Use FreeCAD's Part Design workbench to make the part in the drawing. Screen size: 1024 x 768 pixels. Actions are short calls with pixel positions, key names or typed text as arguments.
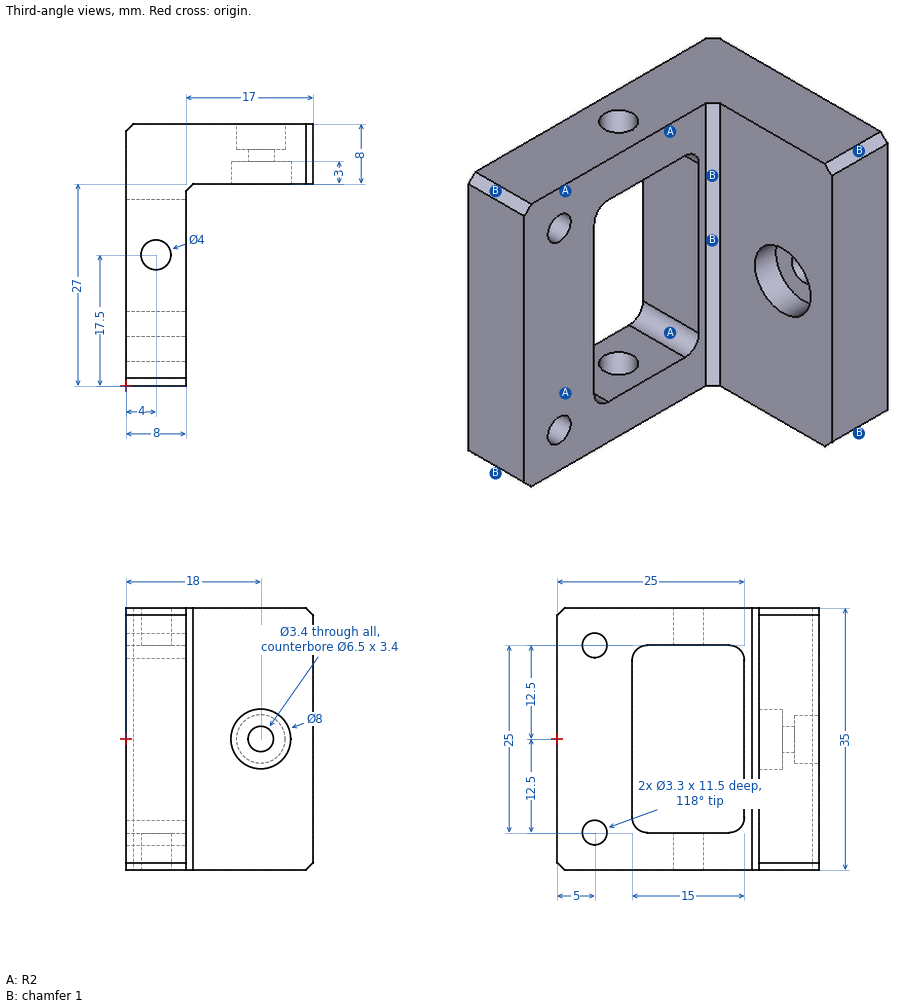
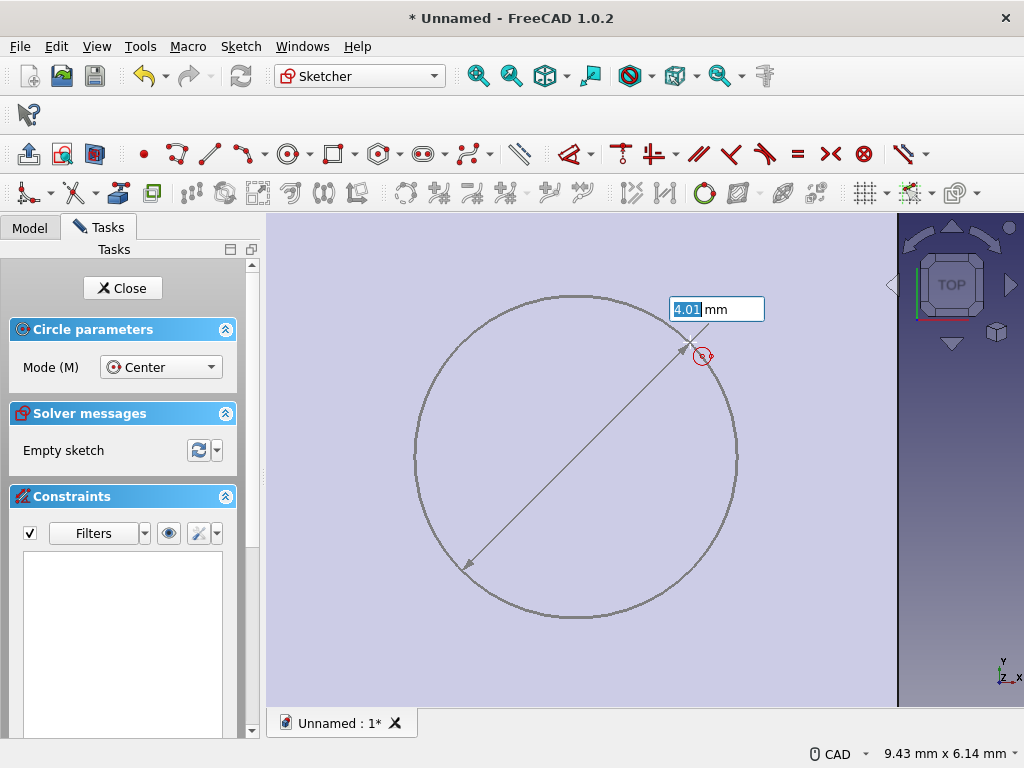
text(4)
key(Return)
key(Escape)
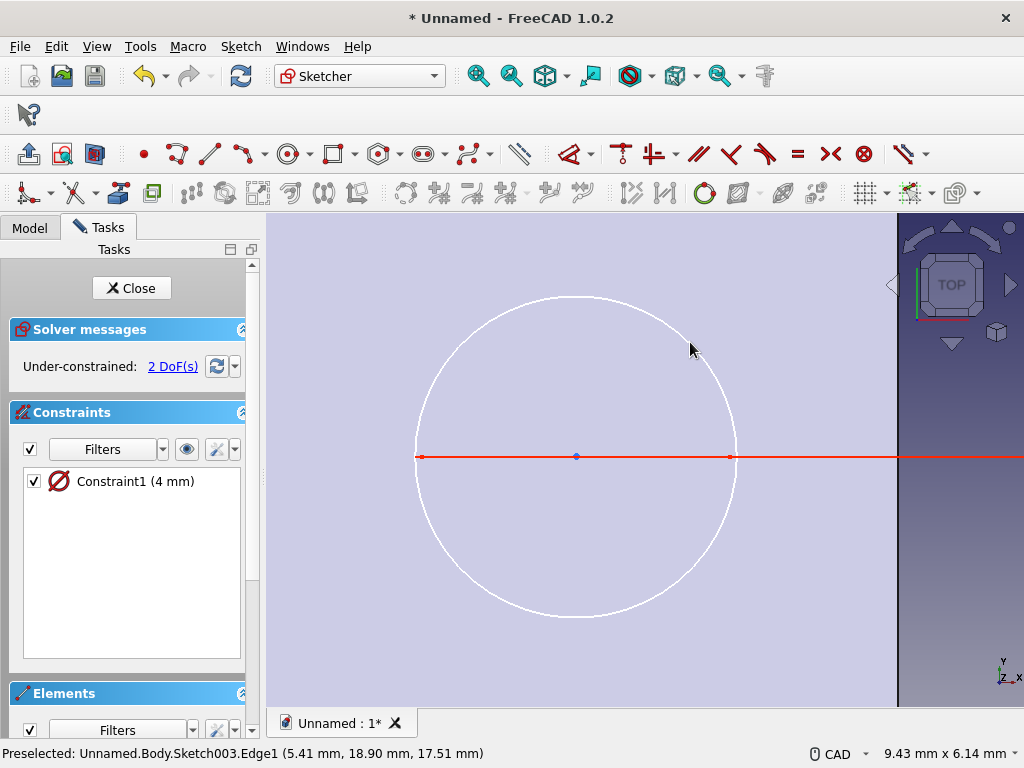
key(d)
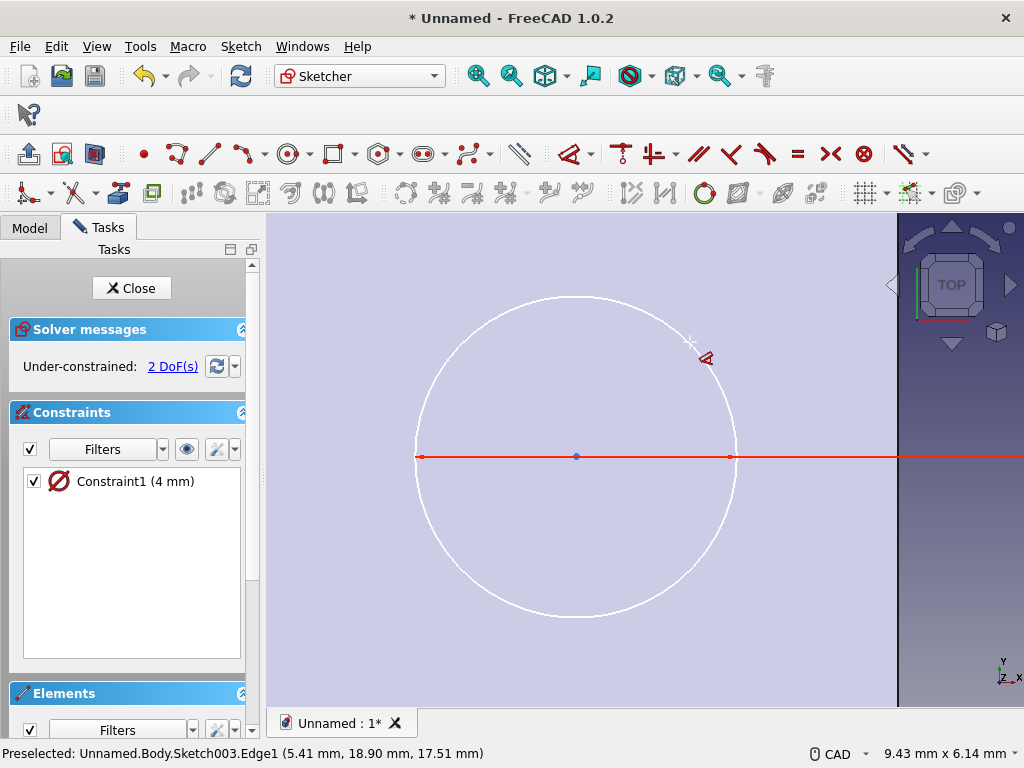
click(576, 457)
click(435, 423)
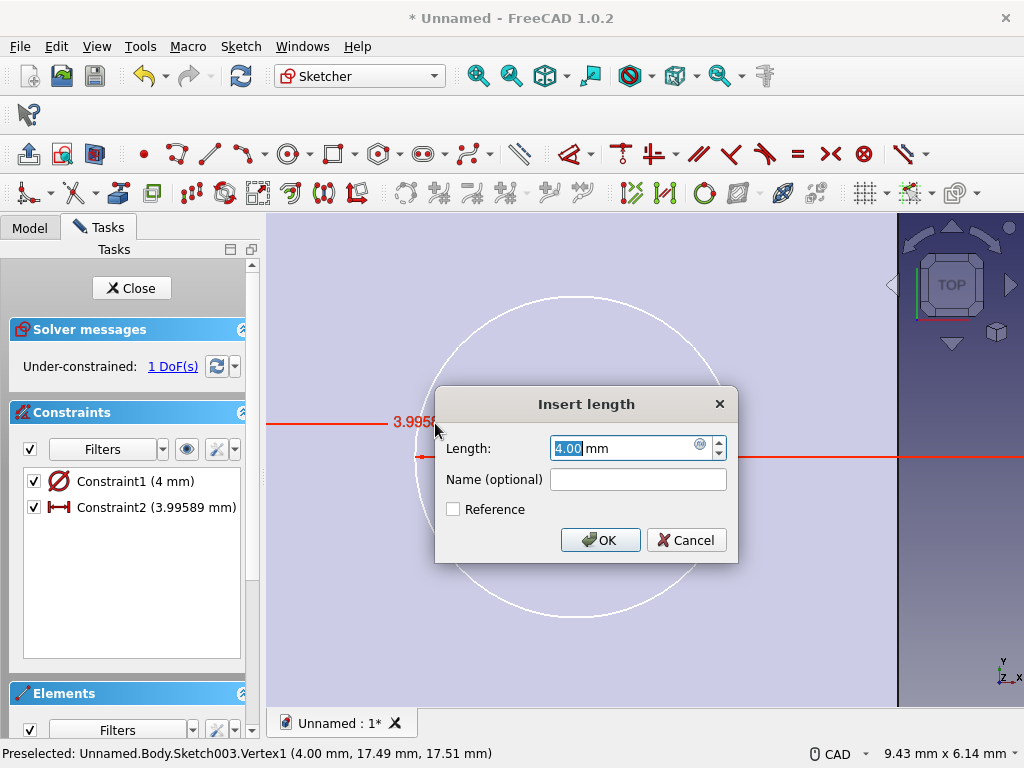
text(4)
key(Return)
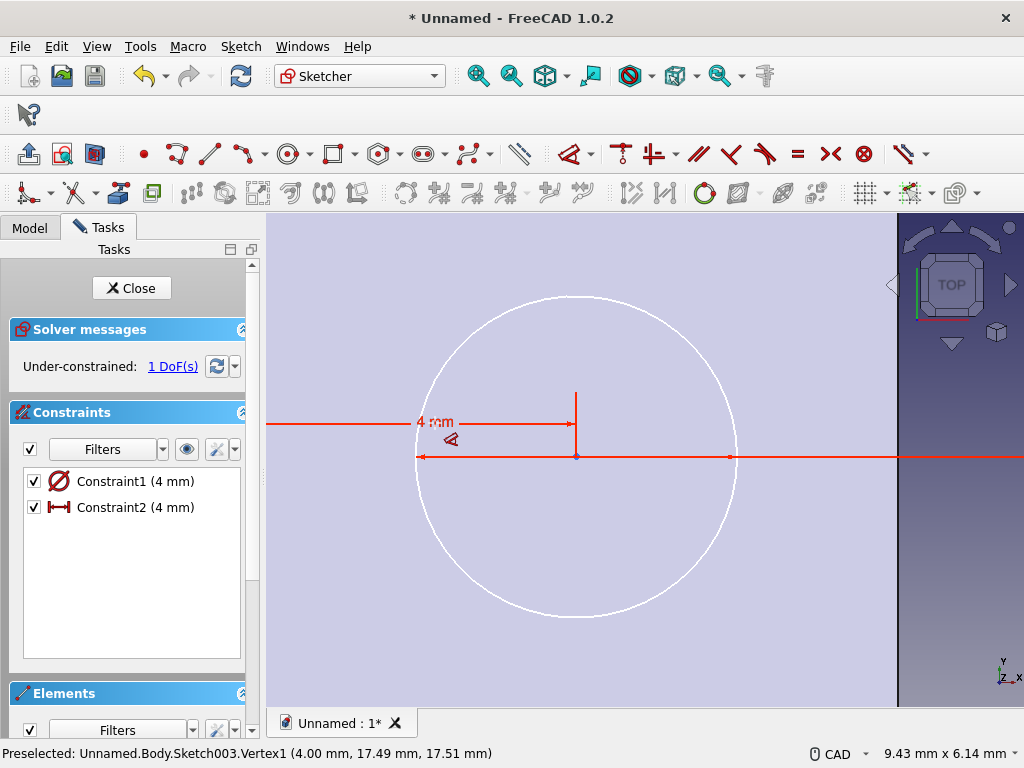
click(576, 457)
click(610, 568)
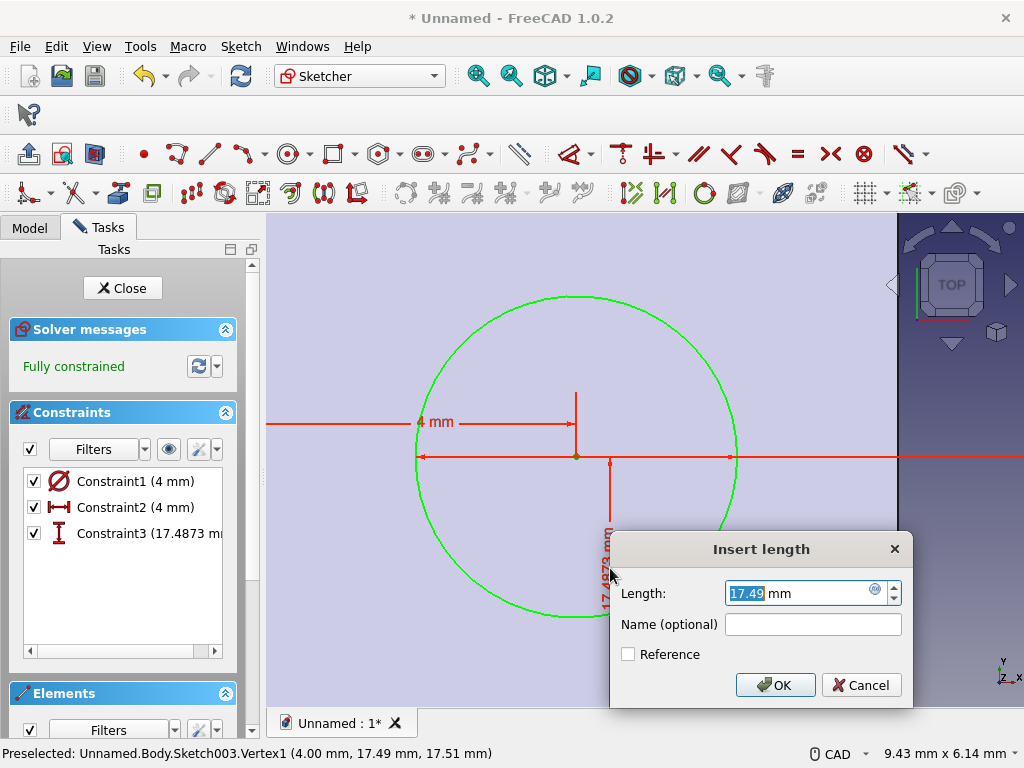
text(17.5)
key(Return)
key(Escape)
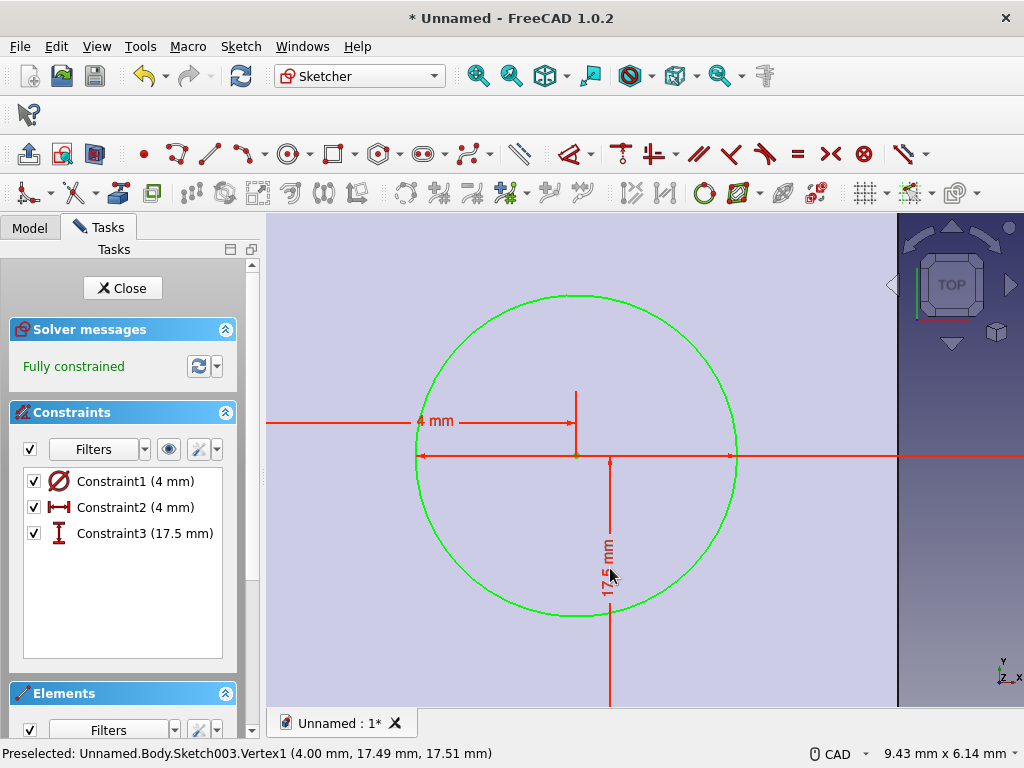
click(123, 288)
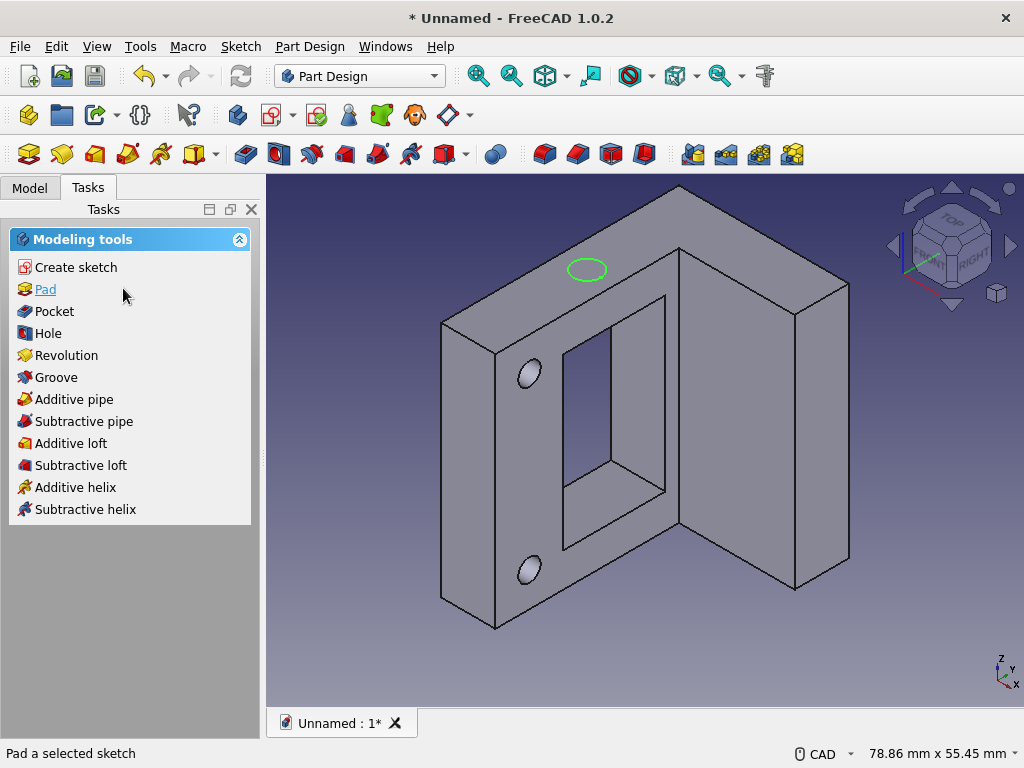
click(246, 154)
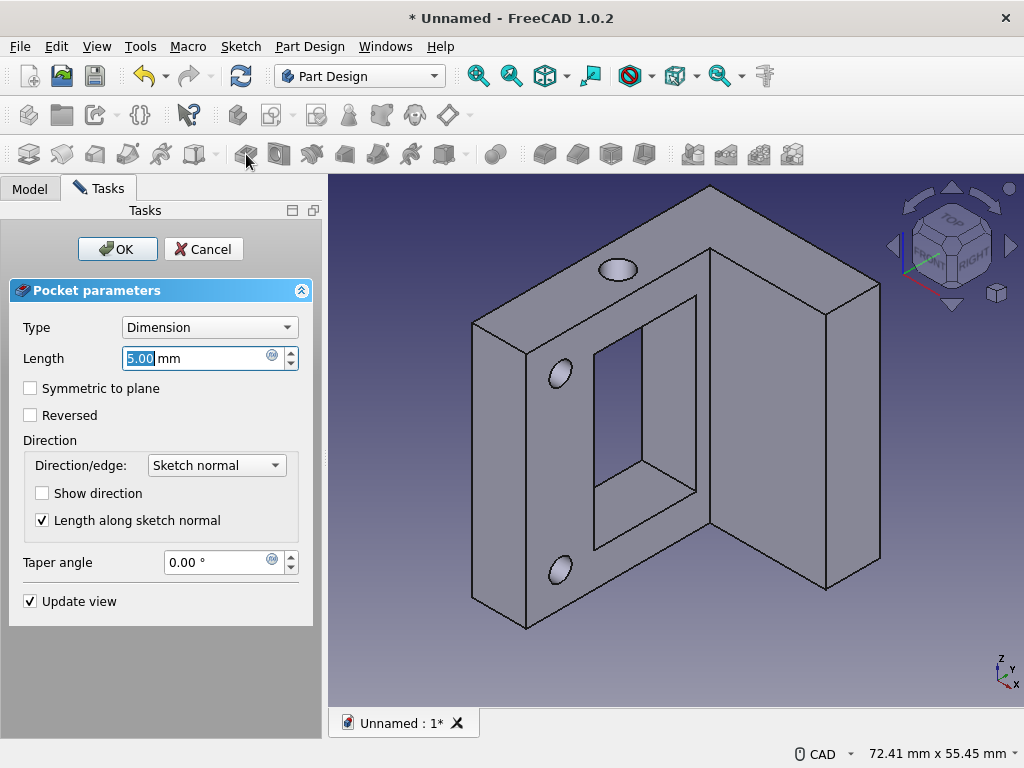
click(210, 328)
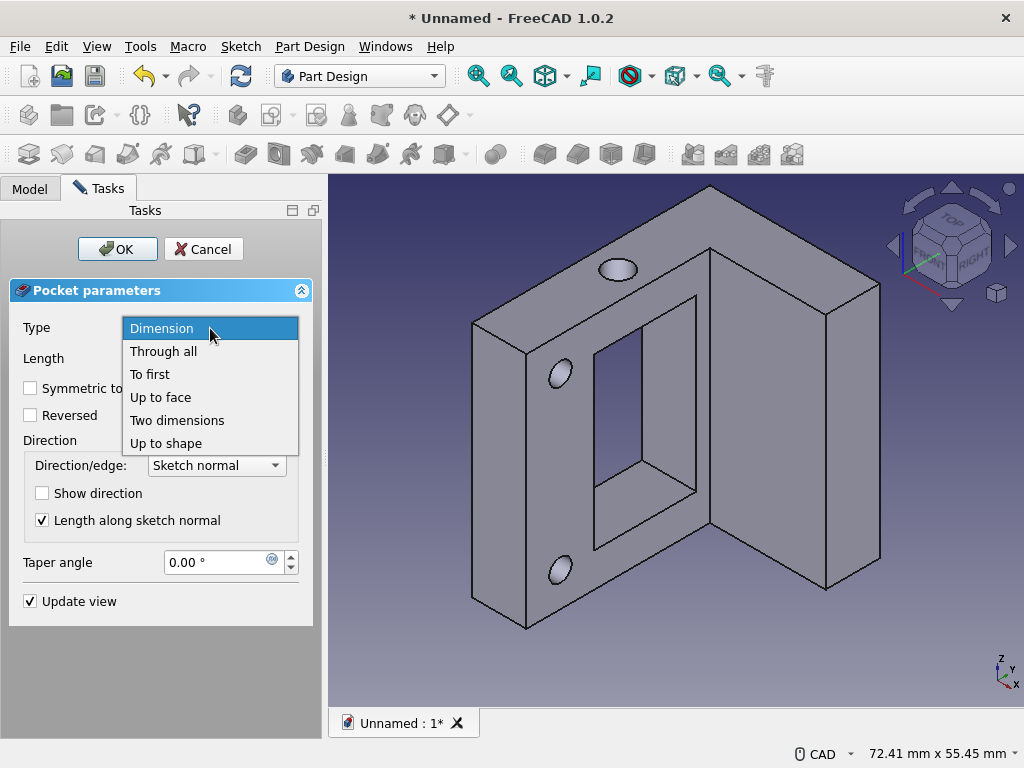
click(208, 352)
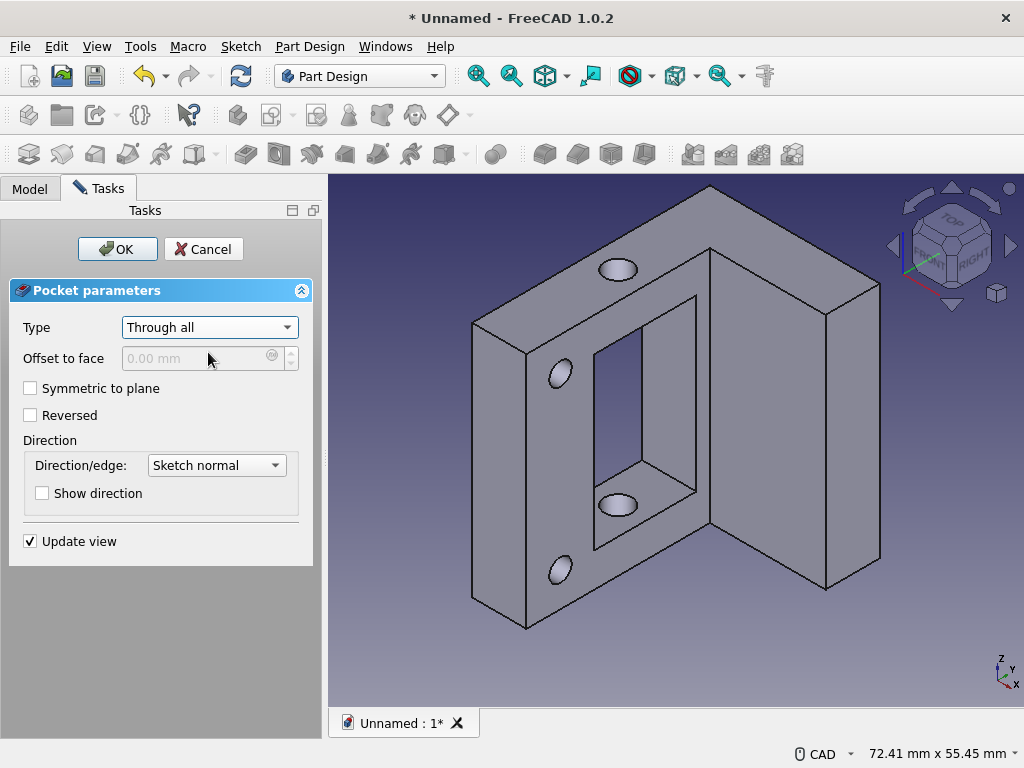
click(118, 249)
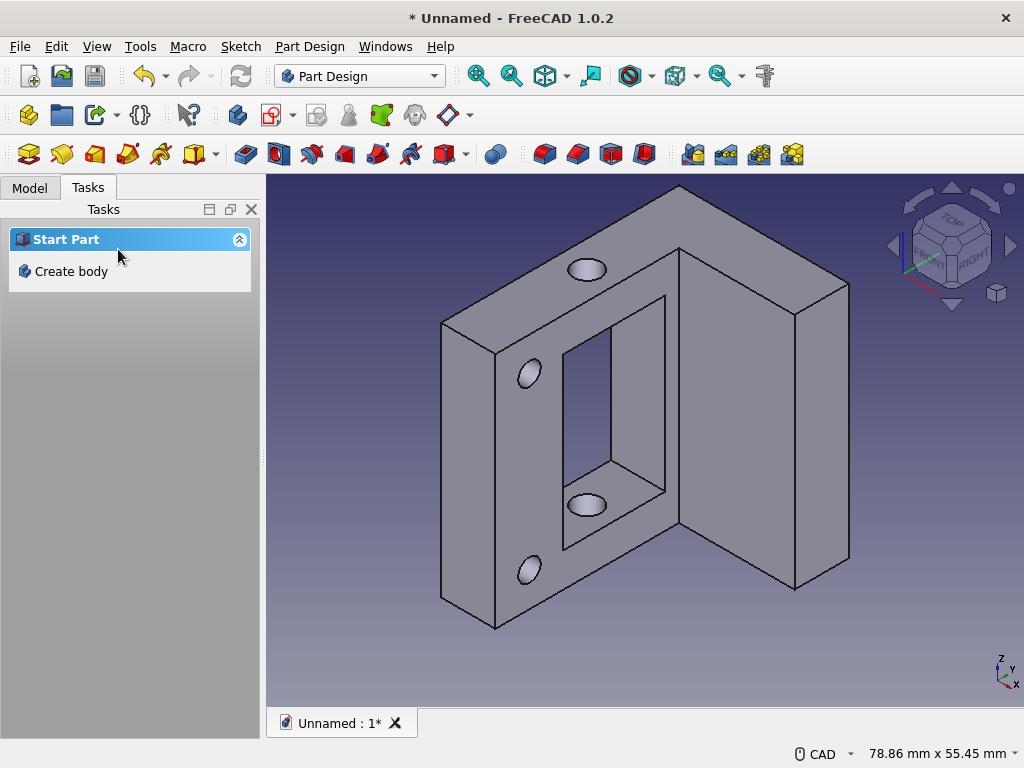
key(2)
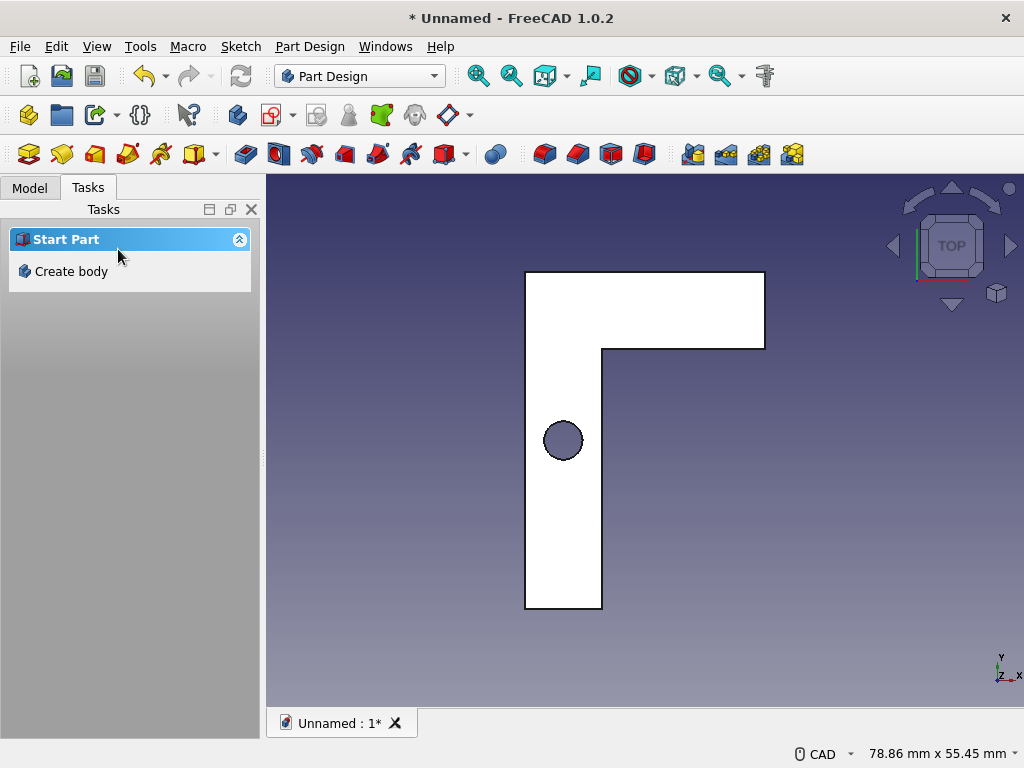
key(0)